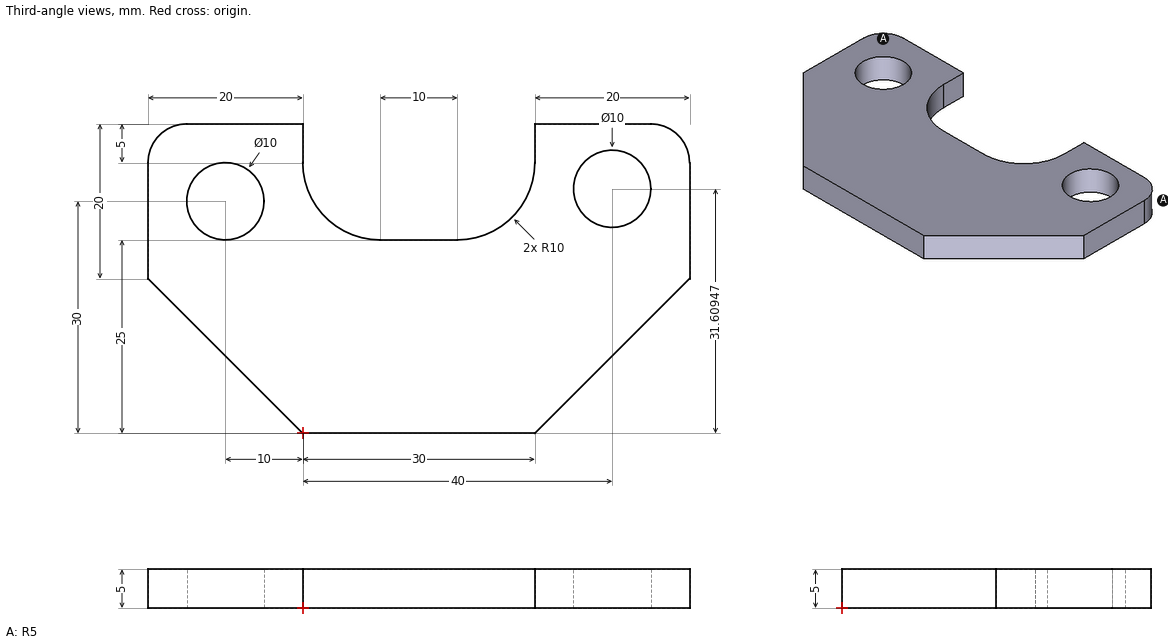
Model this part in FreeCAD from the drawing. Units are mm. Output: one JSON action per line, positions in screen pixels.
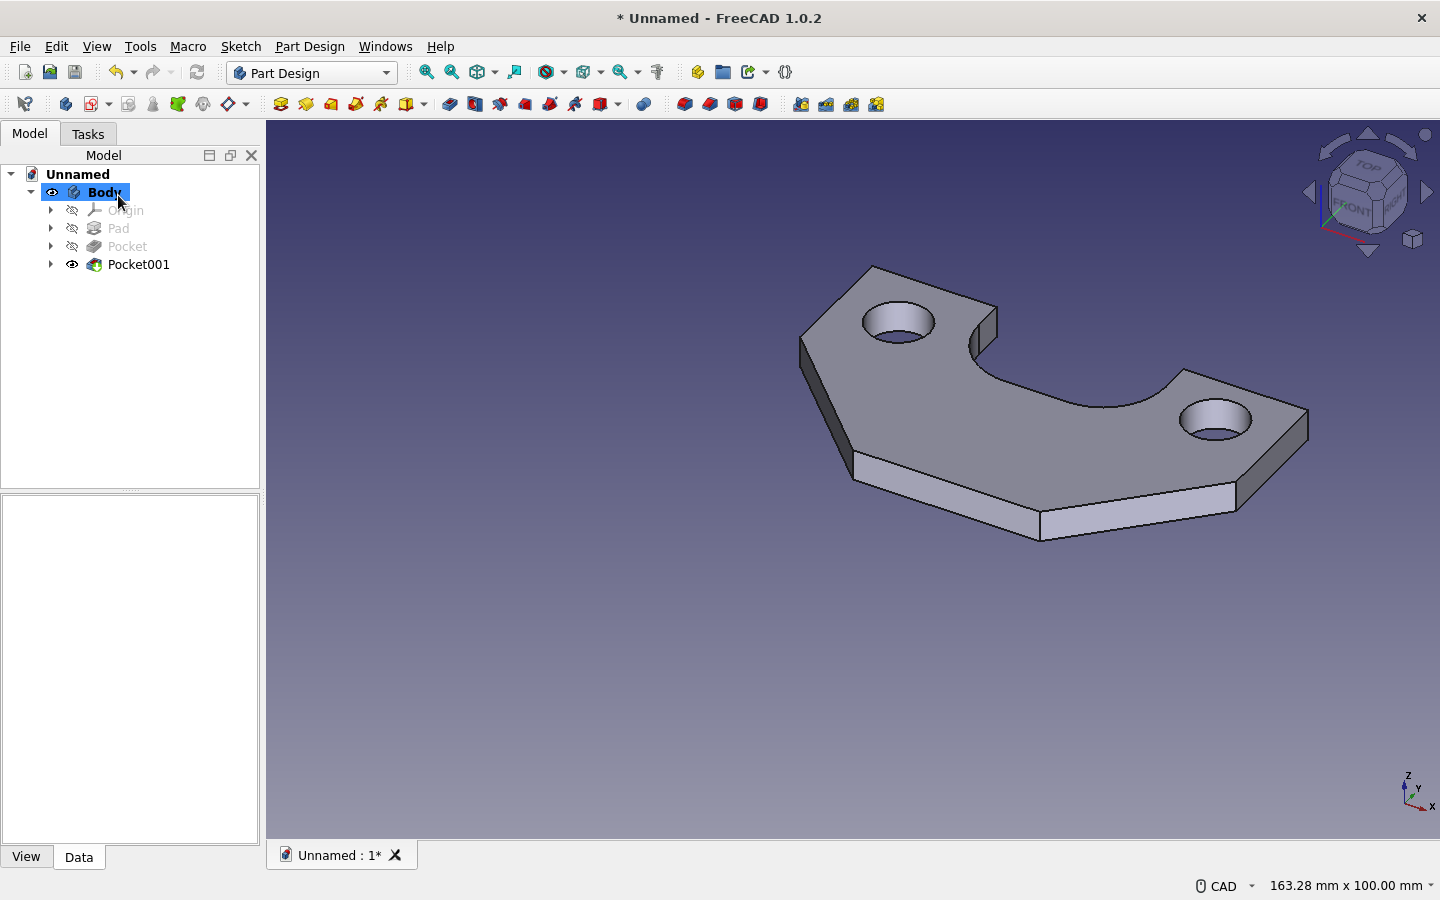
{"action": "key", "text": "0"}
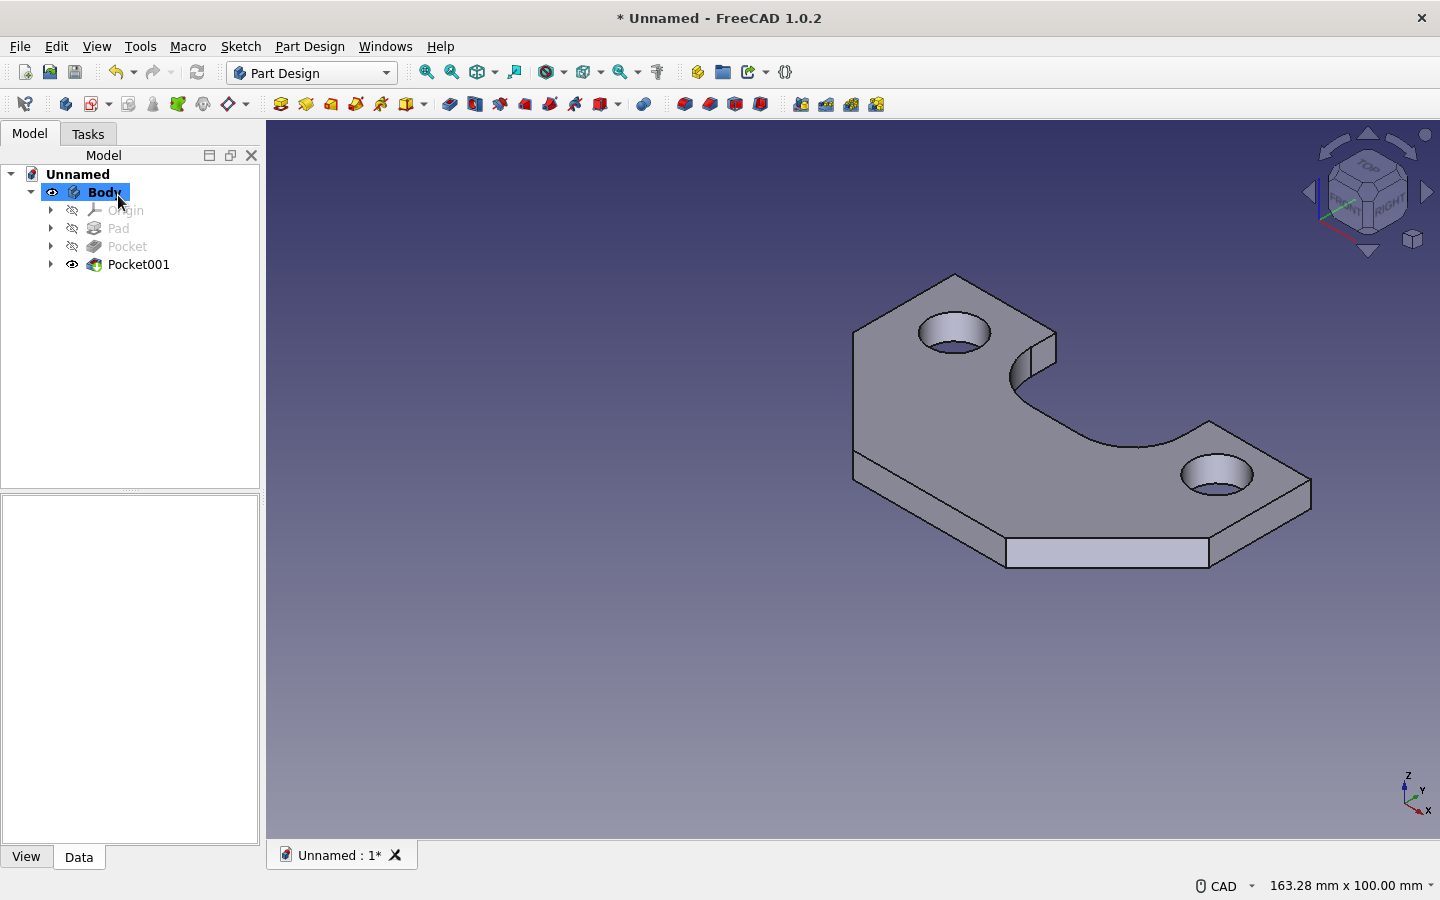
{"action": "key", "text": "2"}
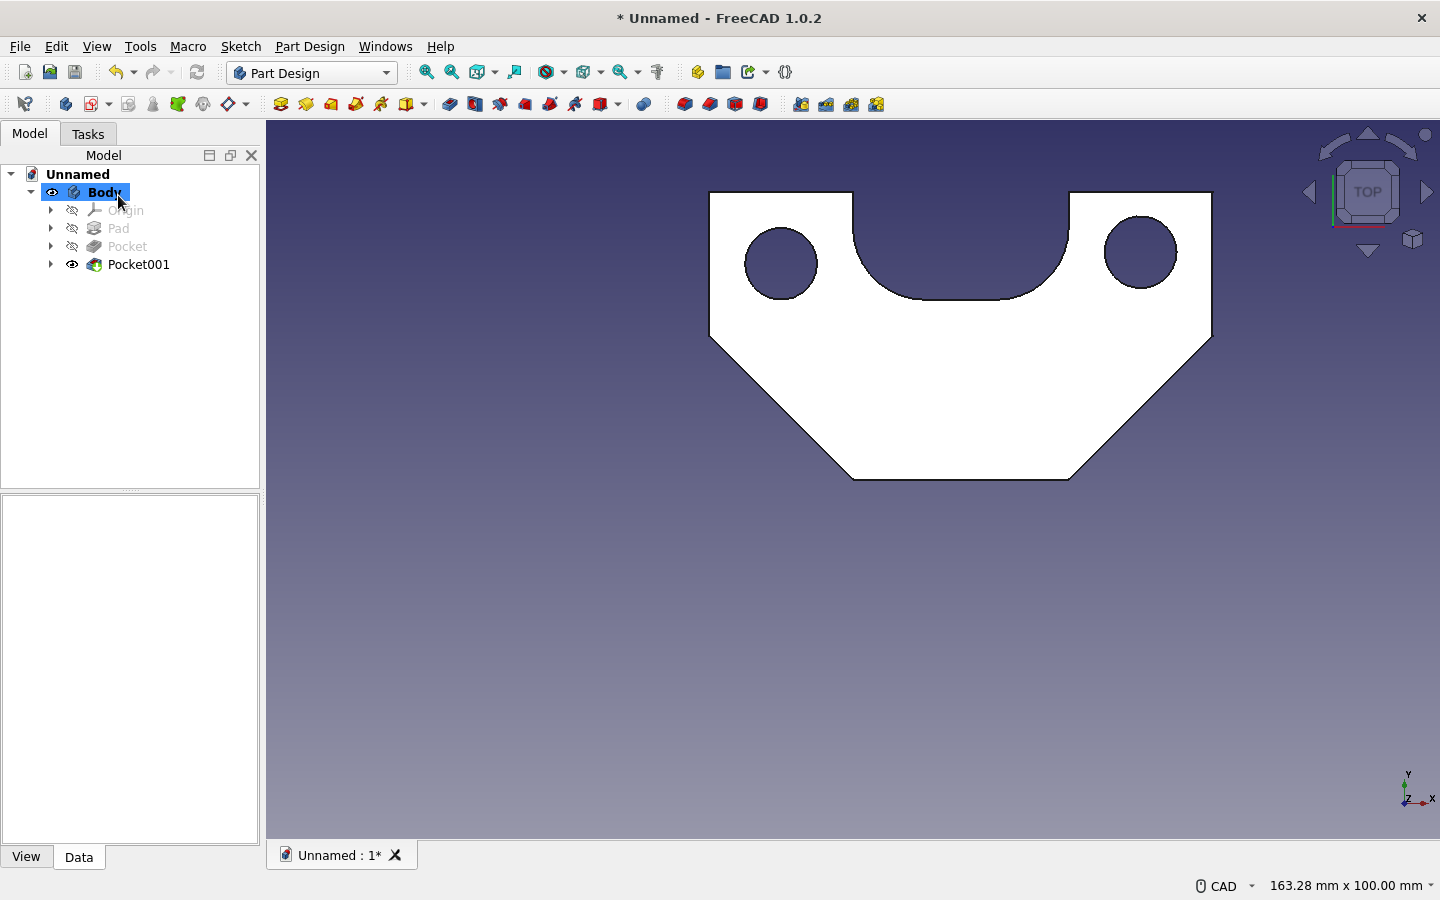
{"action": "left_click", "coordinate": [427, 72]}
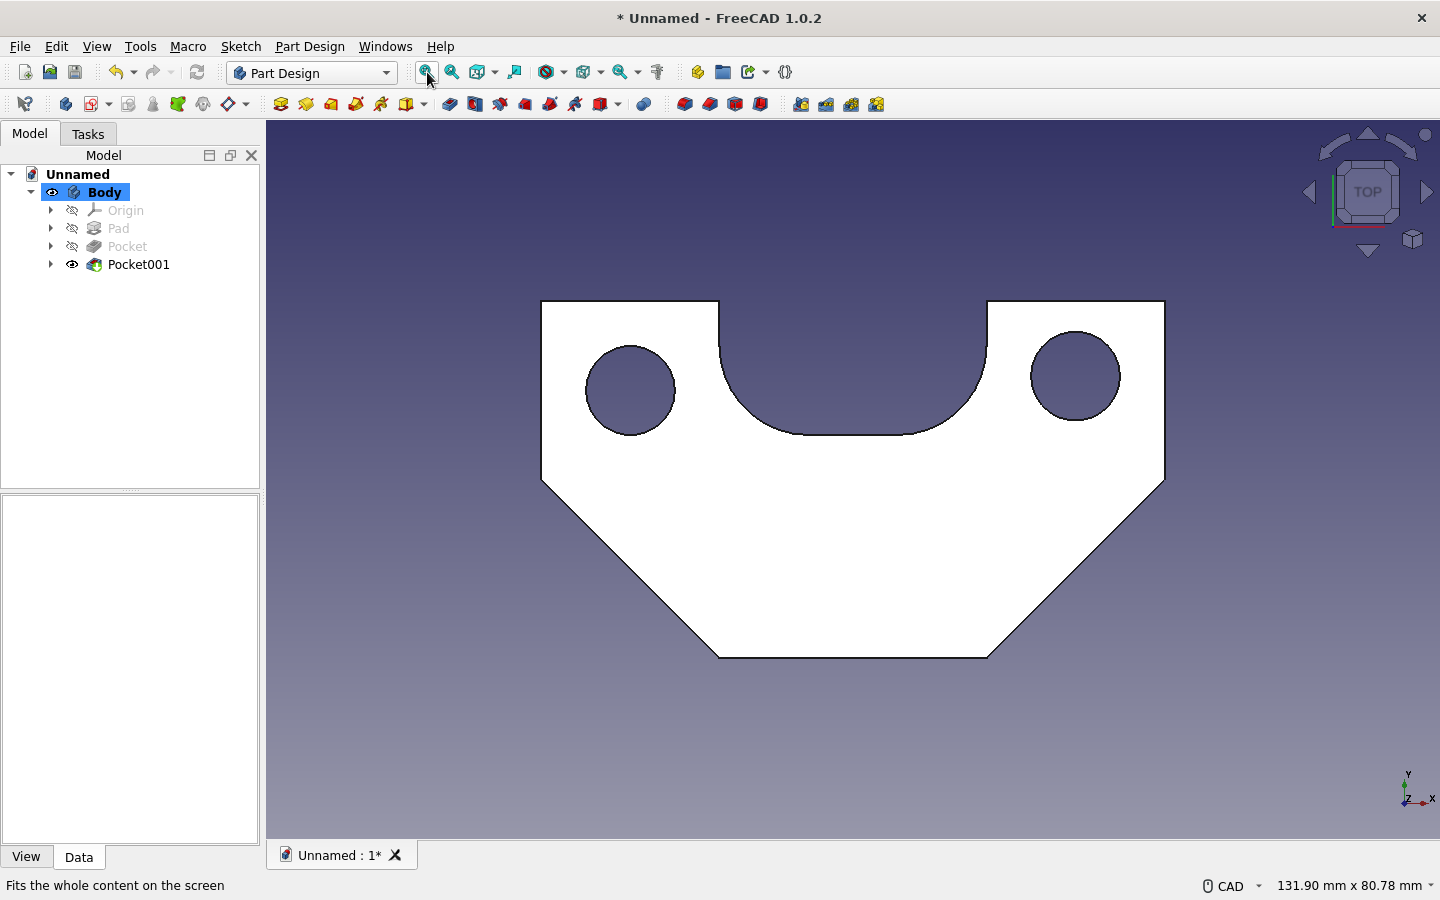
{"action": "key", "text": "1"}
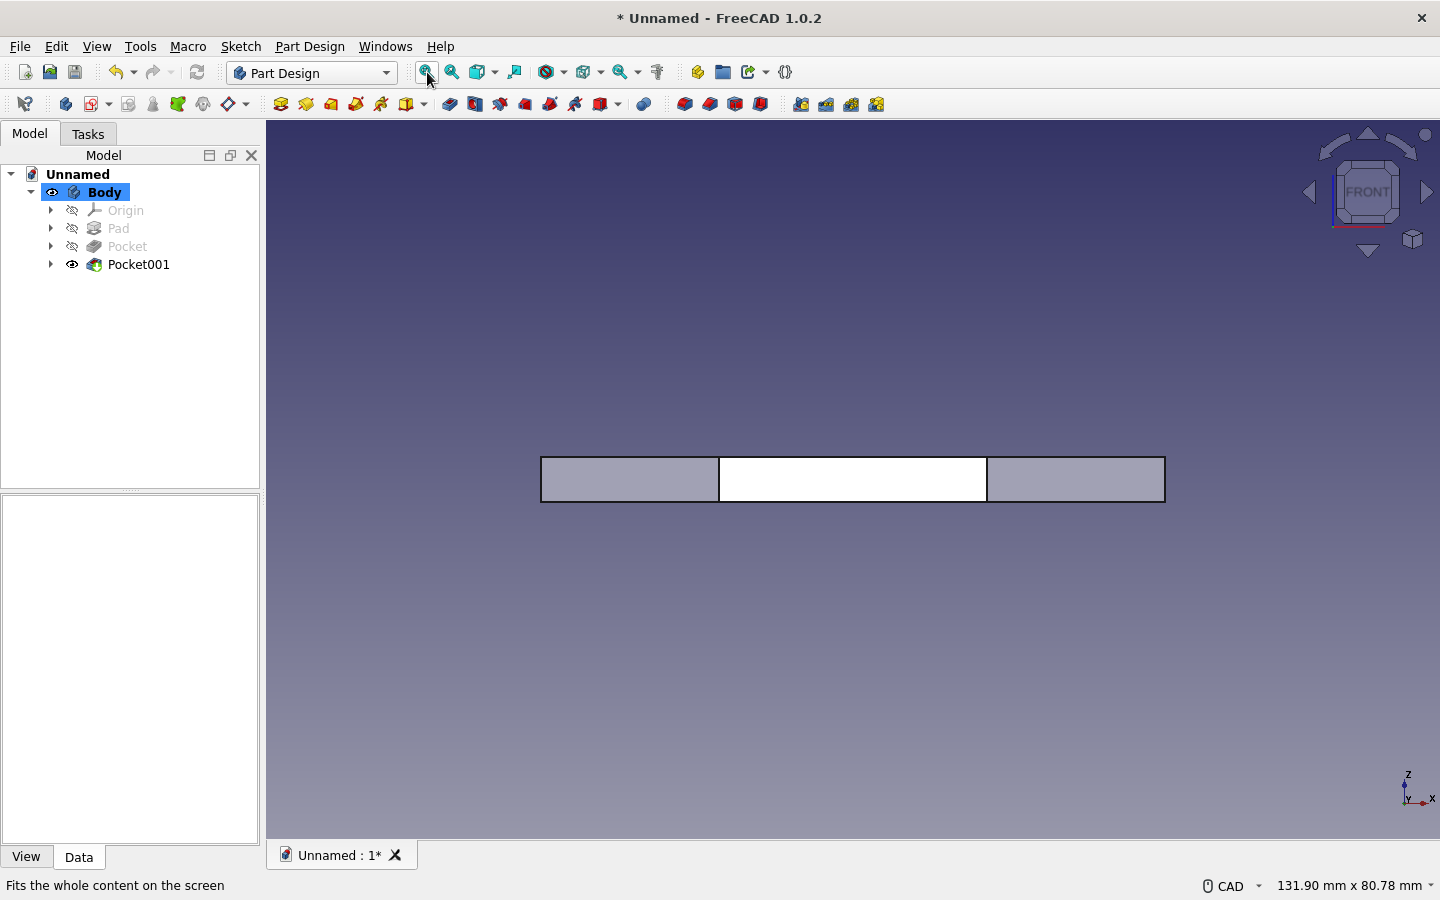
{"action": "key", "text": "3"}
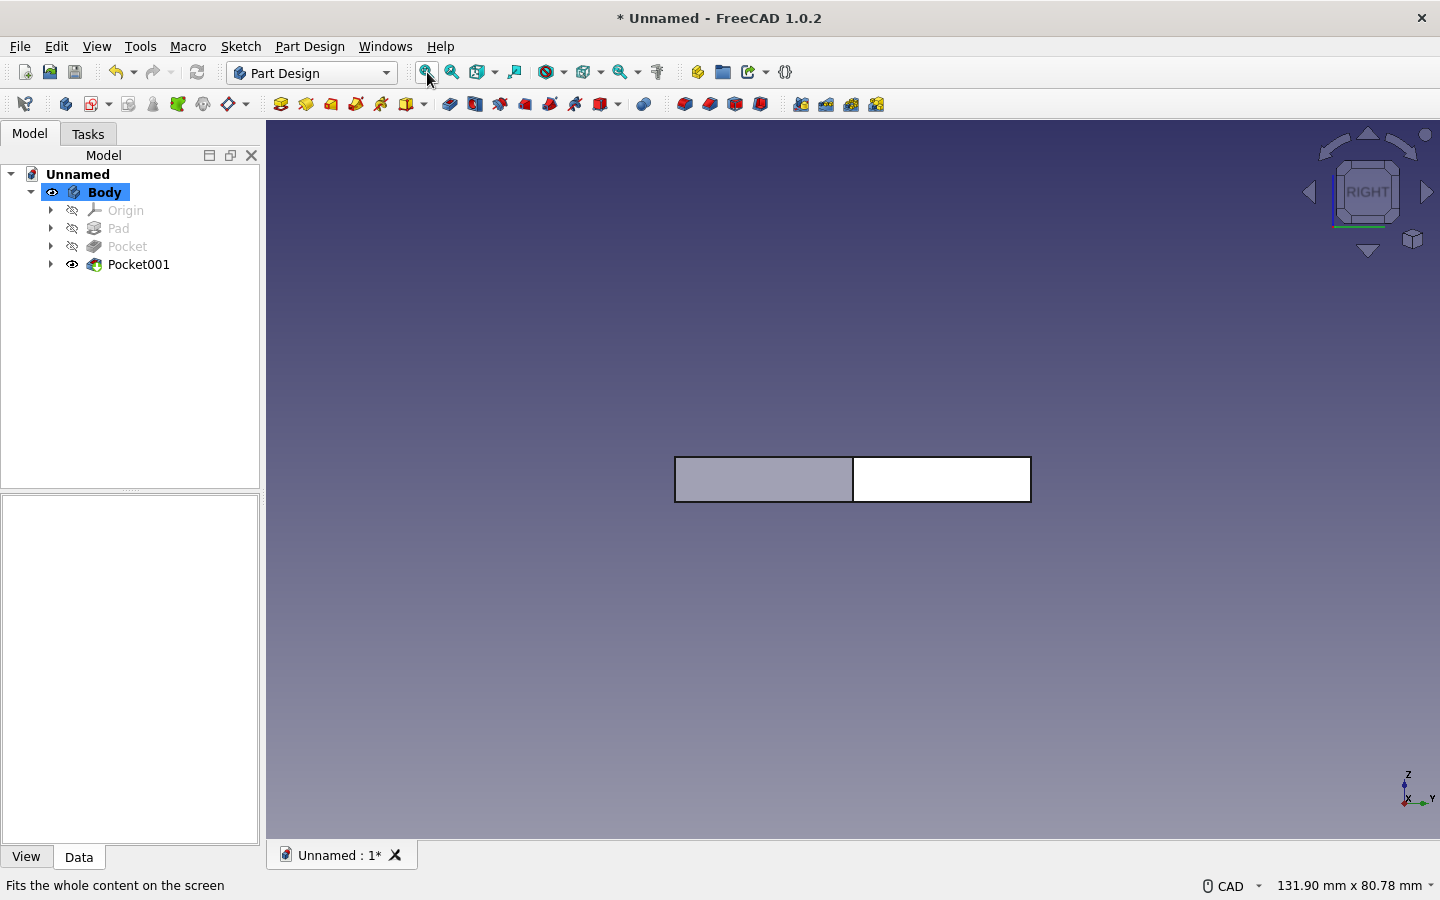
{"action": "left_click", "coordinate": [427, 72]}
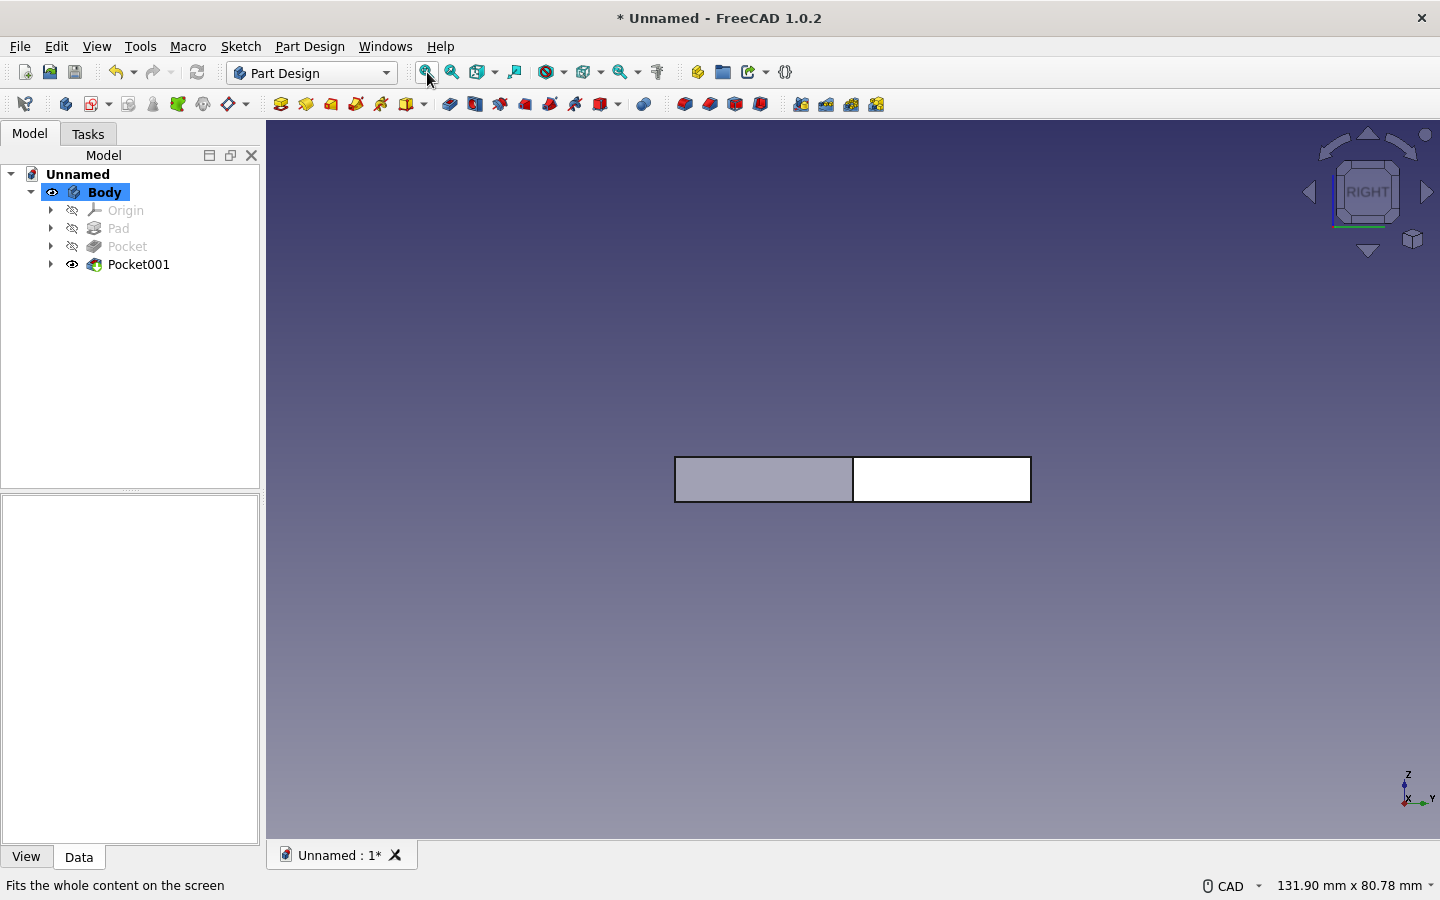
{"action": "left_click", "coordinate": [1031, 478]}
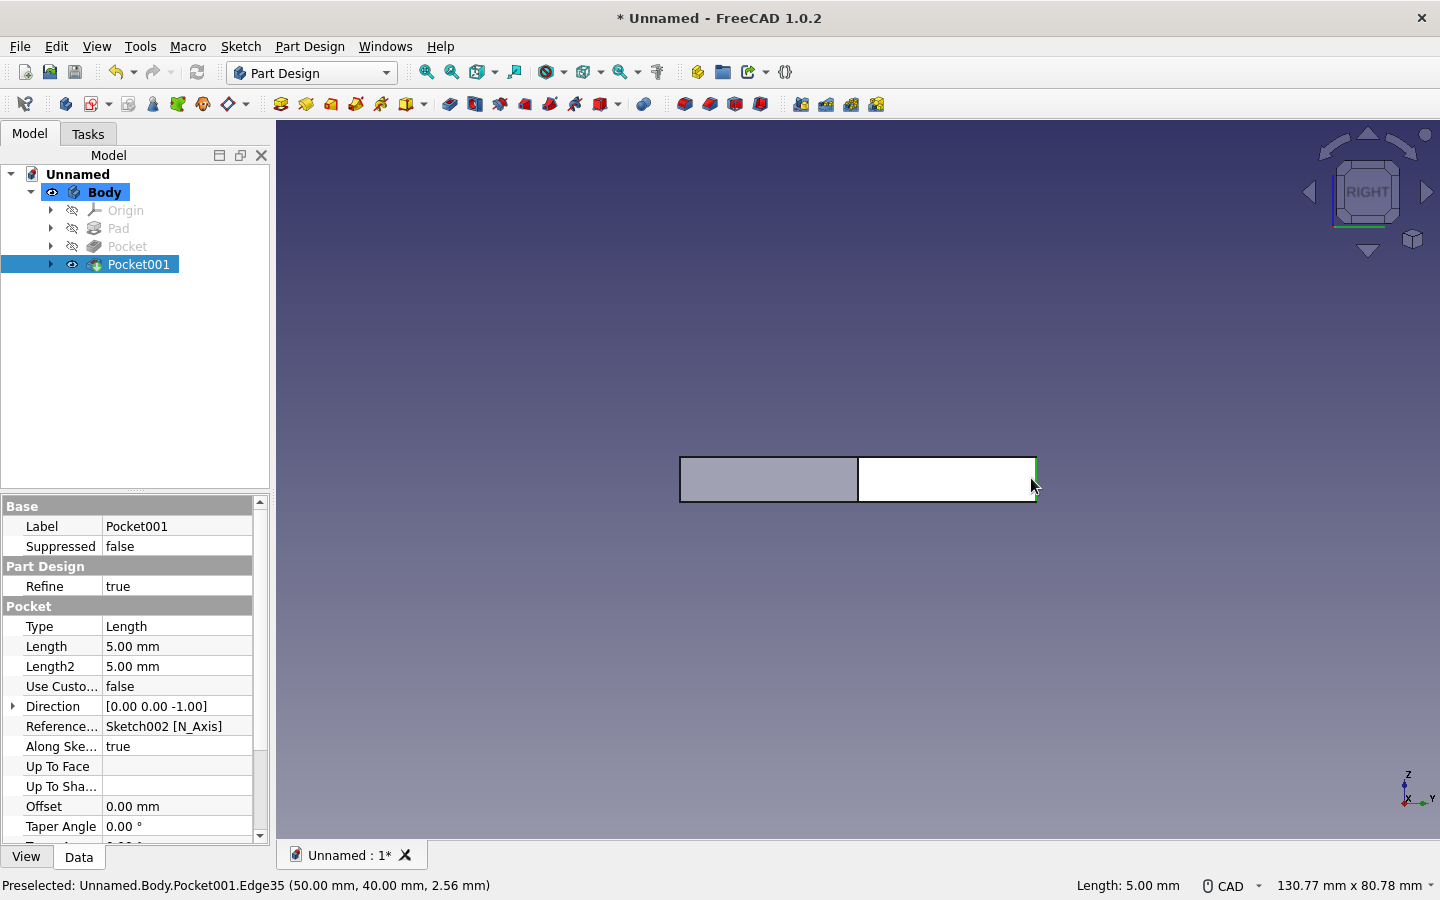
{"action": "key", "text": "5"}